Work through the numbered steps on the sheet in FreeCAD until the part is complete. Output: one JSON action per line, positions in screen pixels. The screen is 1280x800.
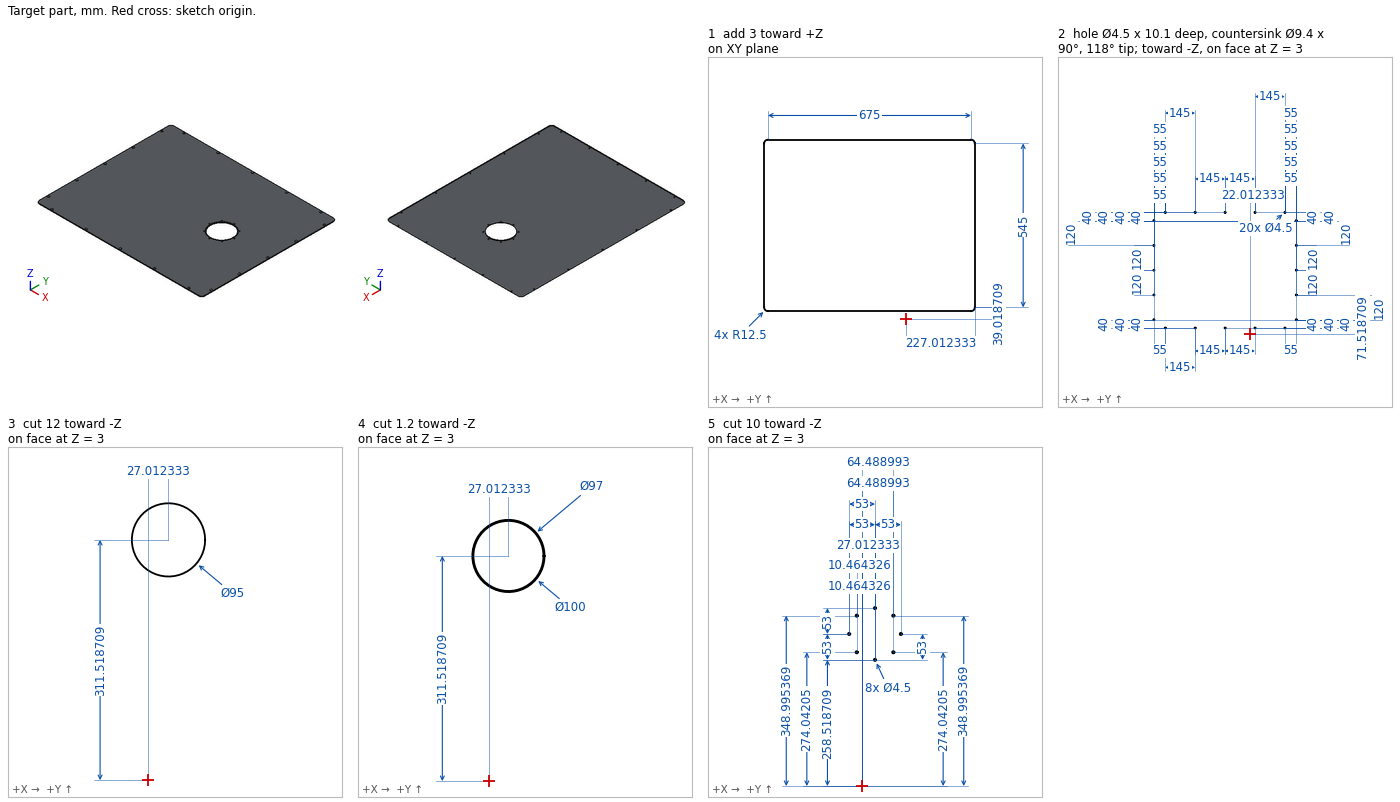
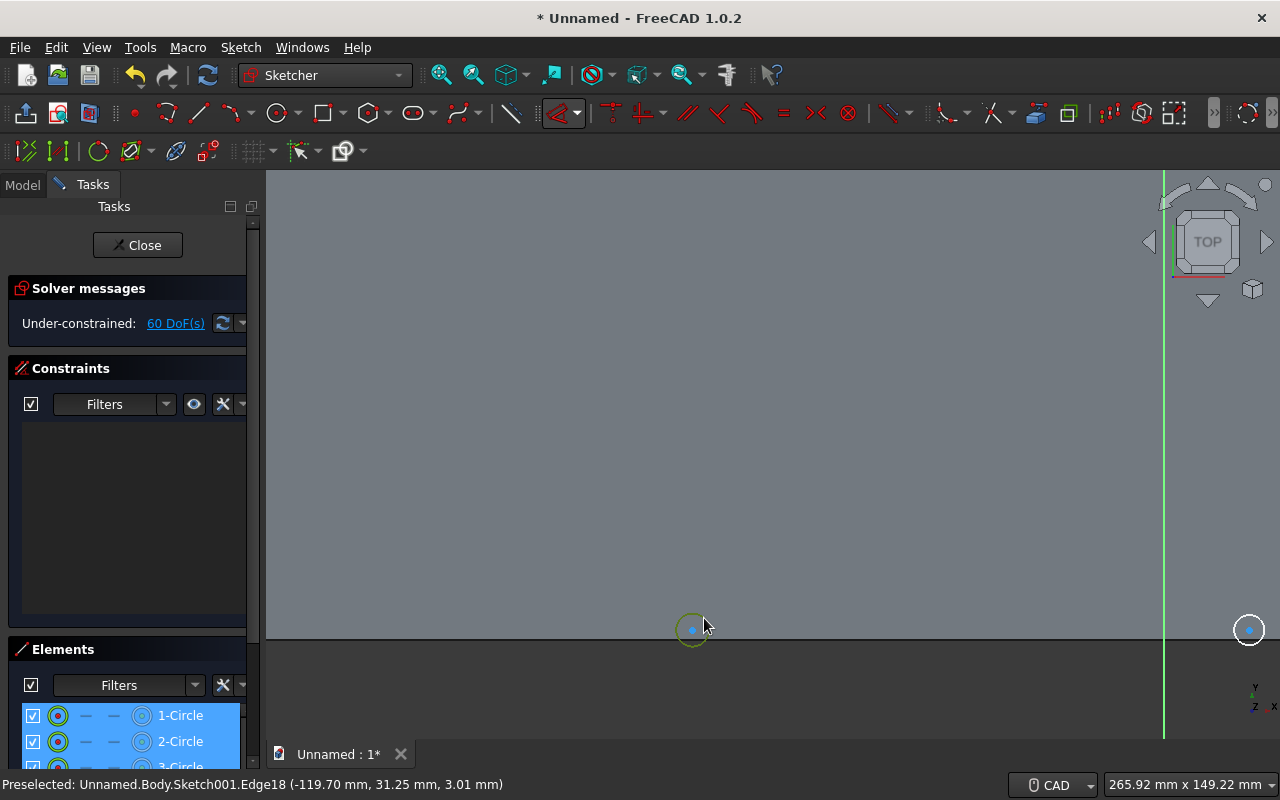
{"action": "scroll", "coordinate": [706, 622], "scroll_direction": "down", "scroll_amount": 9}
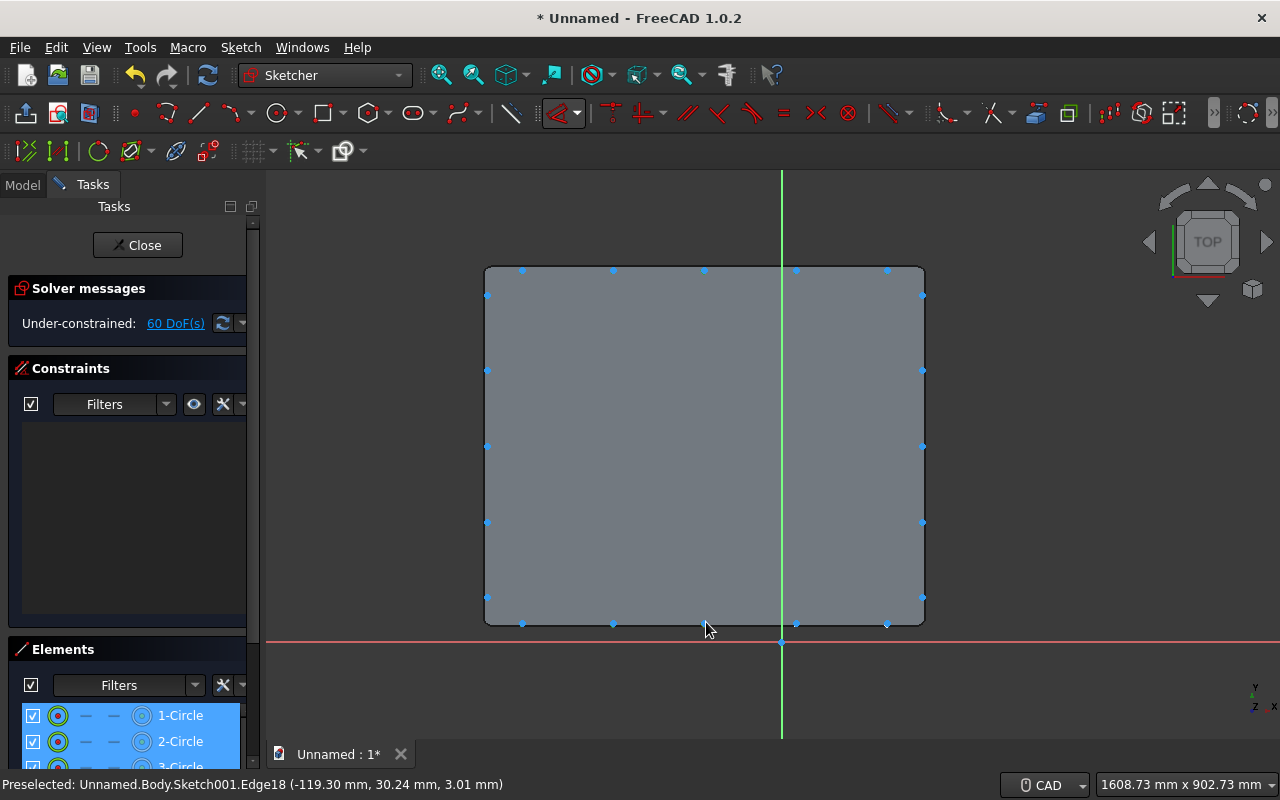
{"action": "scroll", "coordinate": [798, 622], "scroll_direction": "up", "scroll_amount": 9}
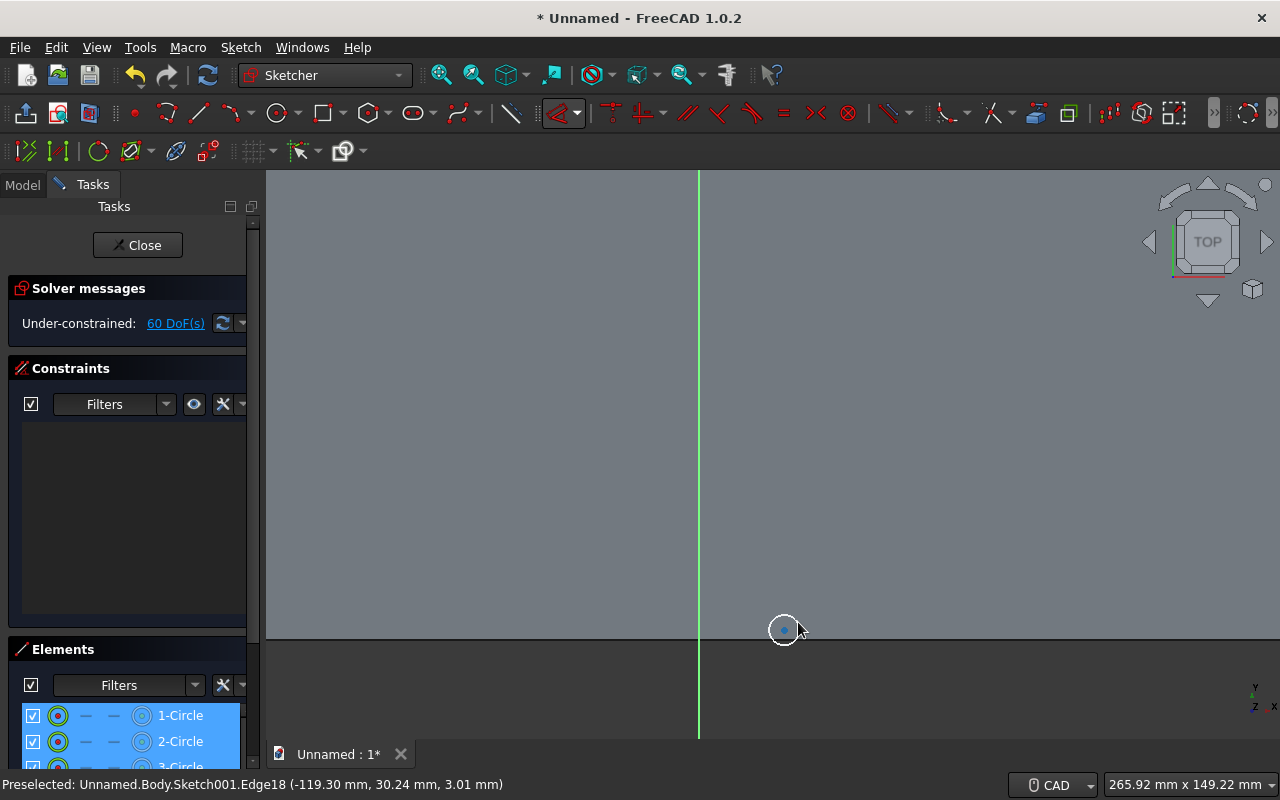
{"action": "left_click", "coordinate": [795, 619]}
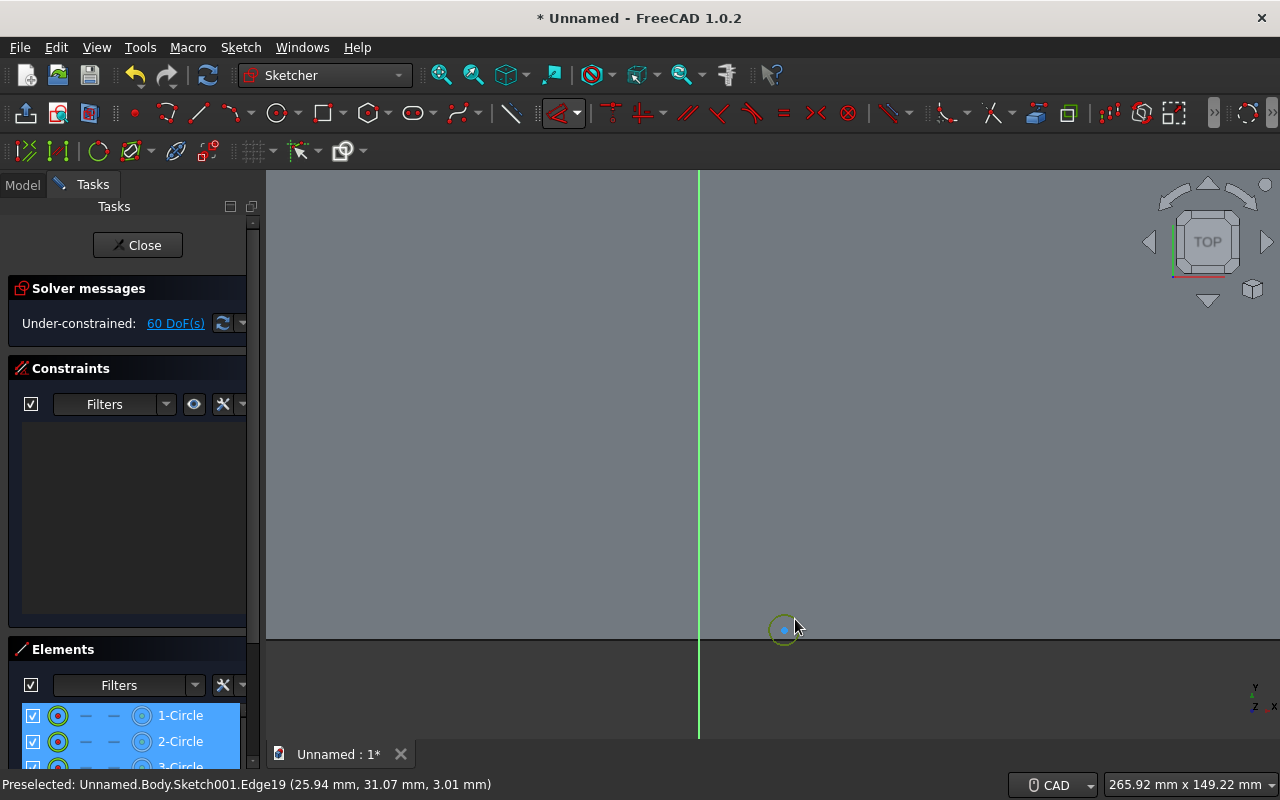
{"action": "scroll", "coordinate": [799, 622], "scroll_direction": "down", "scroll_amount": 9}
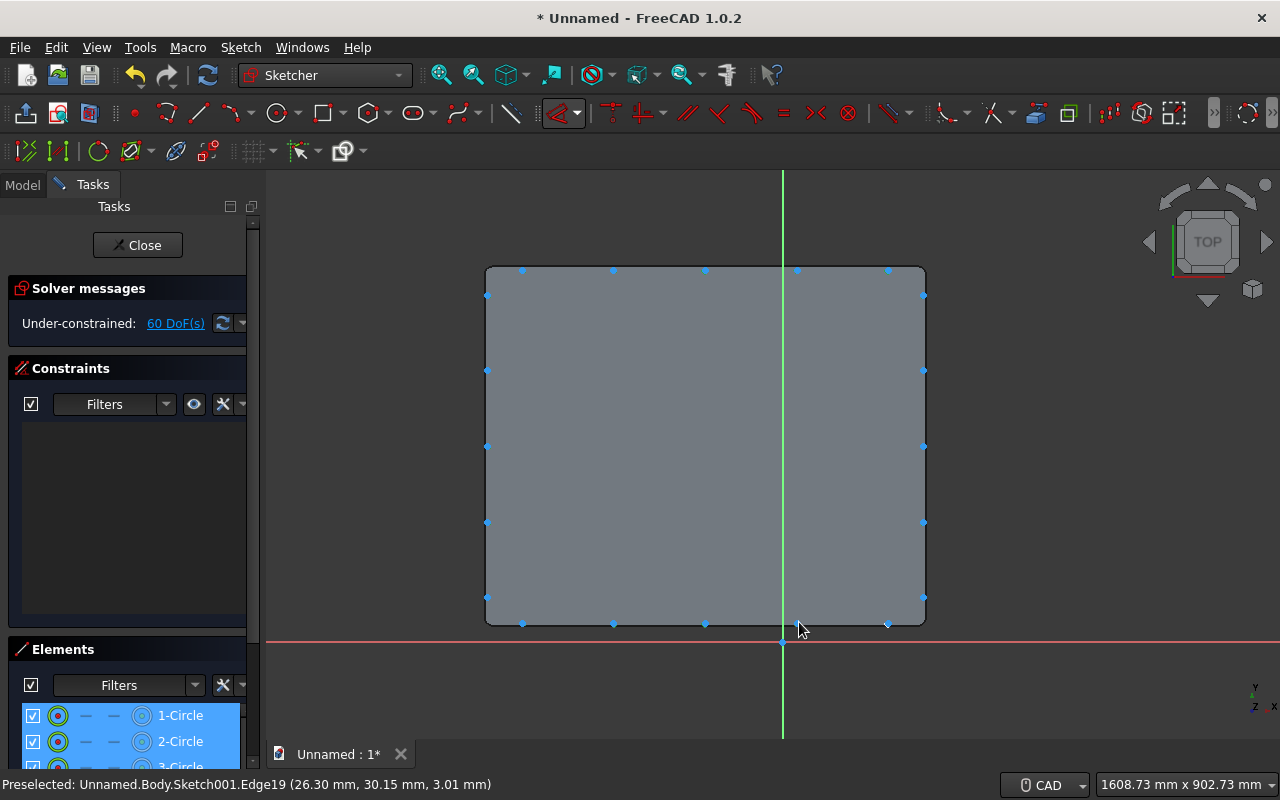
{"action": "scroll", "coordinate": [890, 622], "scroll_direction": "up", "scroll_amount": 9}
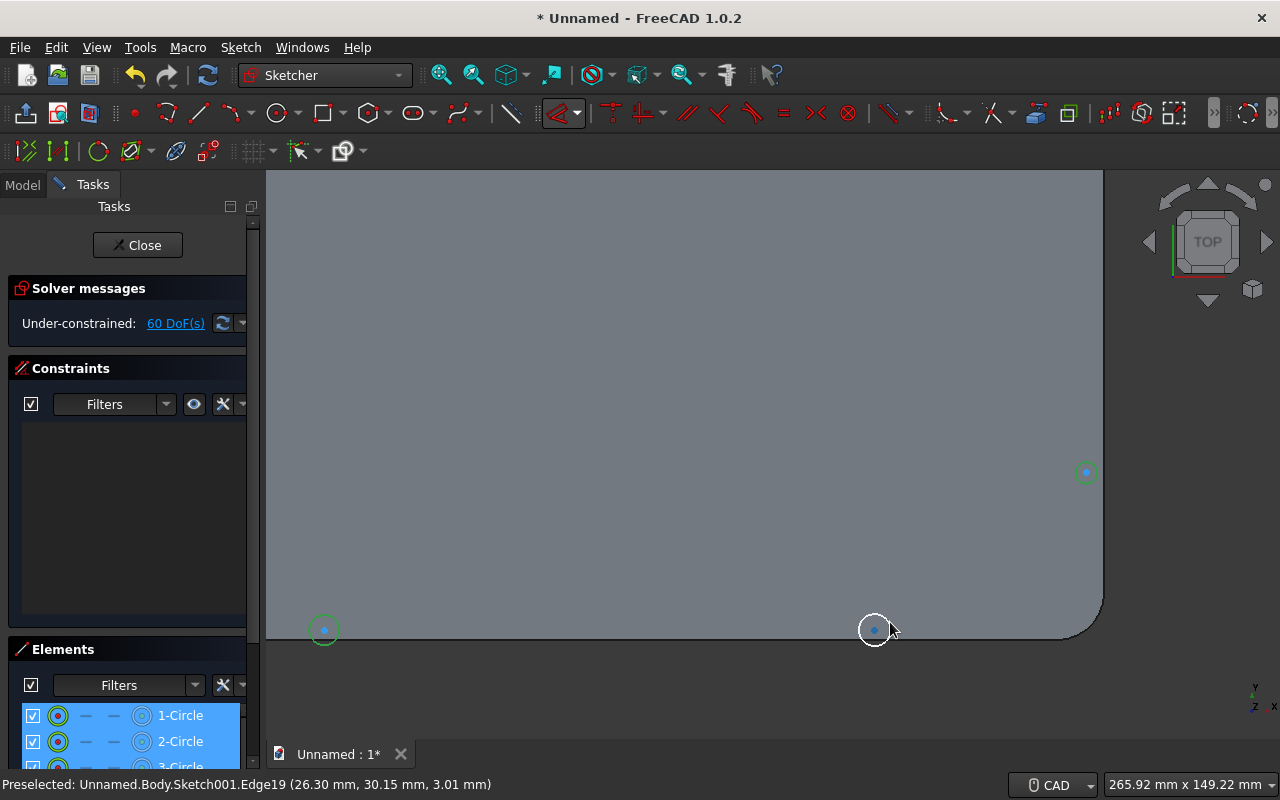
{"action": "left_click", "coordinate": [886, 619]}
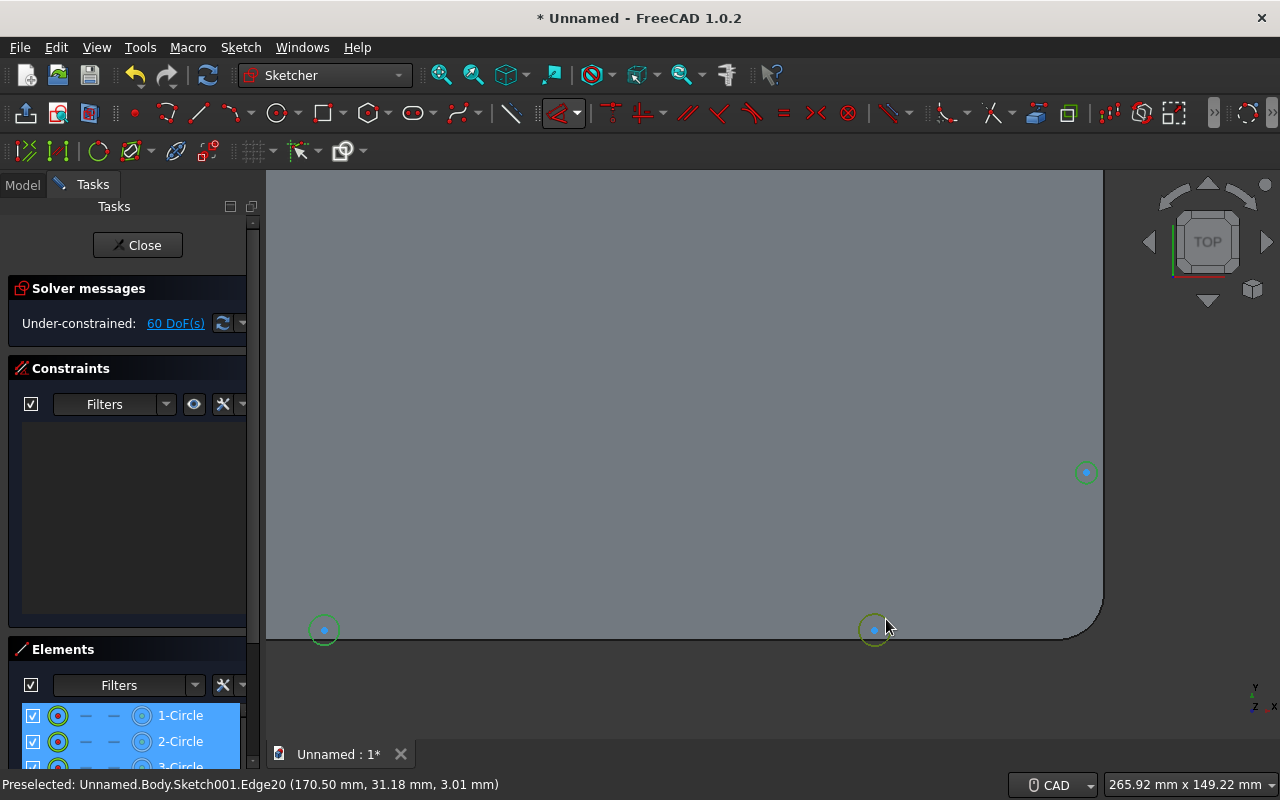
{"action": "left_click", "coordinate": [784, 114]}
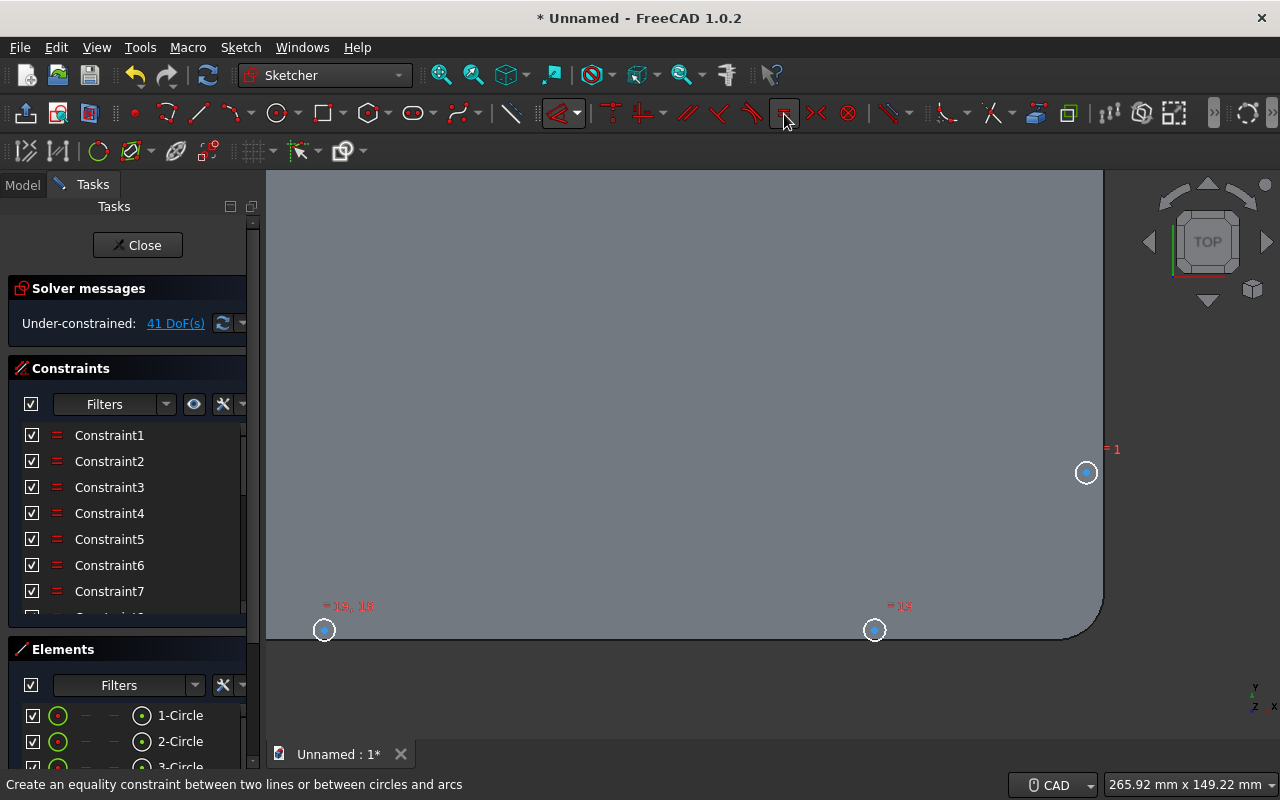
{"action": "scroll", "coordinate": [1094, 465], "scroll_direction": "up", "scroll_amount": 5}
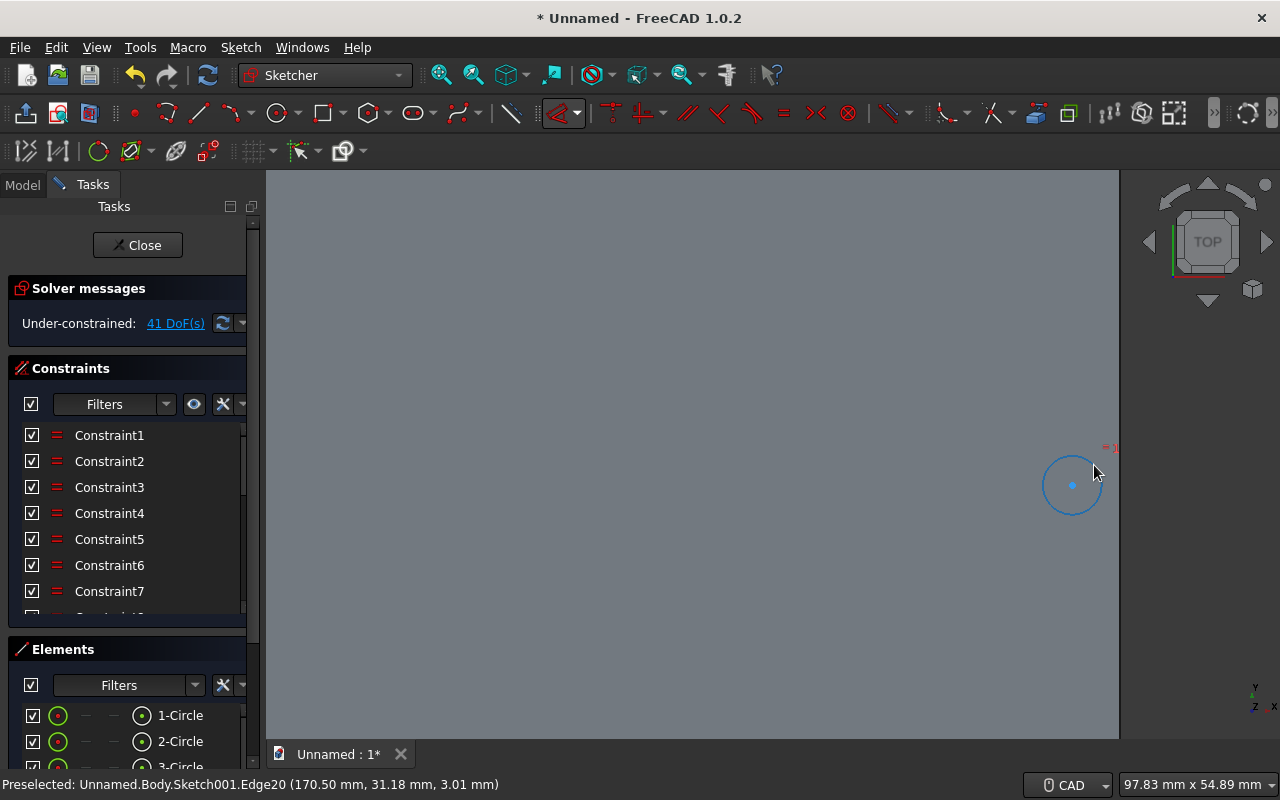
{"action": "left_click", "coordinate": [1093, 464]}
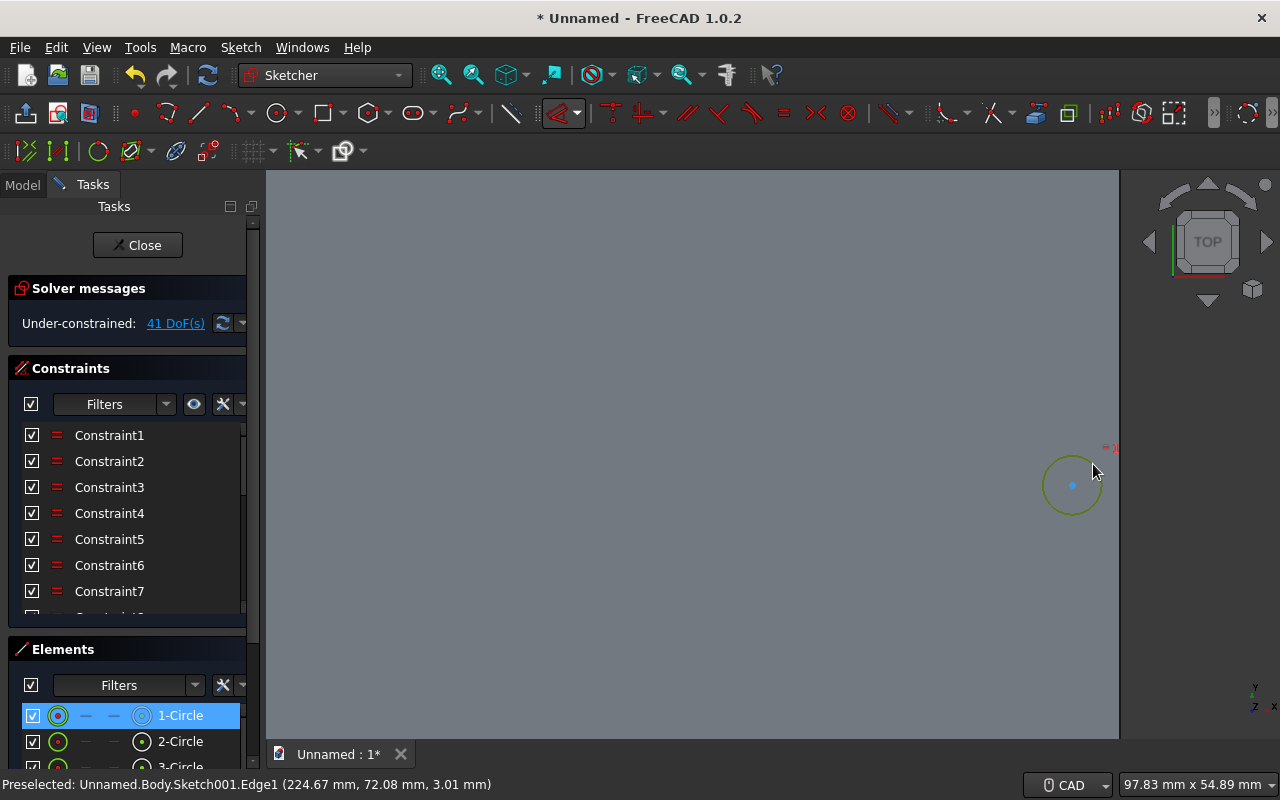
{"action": "key", "text": "k o"}